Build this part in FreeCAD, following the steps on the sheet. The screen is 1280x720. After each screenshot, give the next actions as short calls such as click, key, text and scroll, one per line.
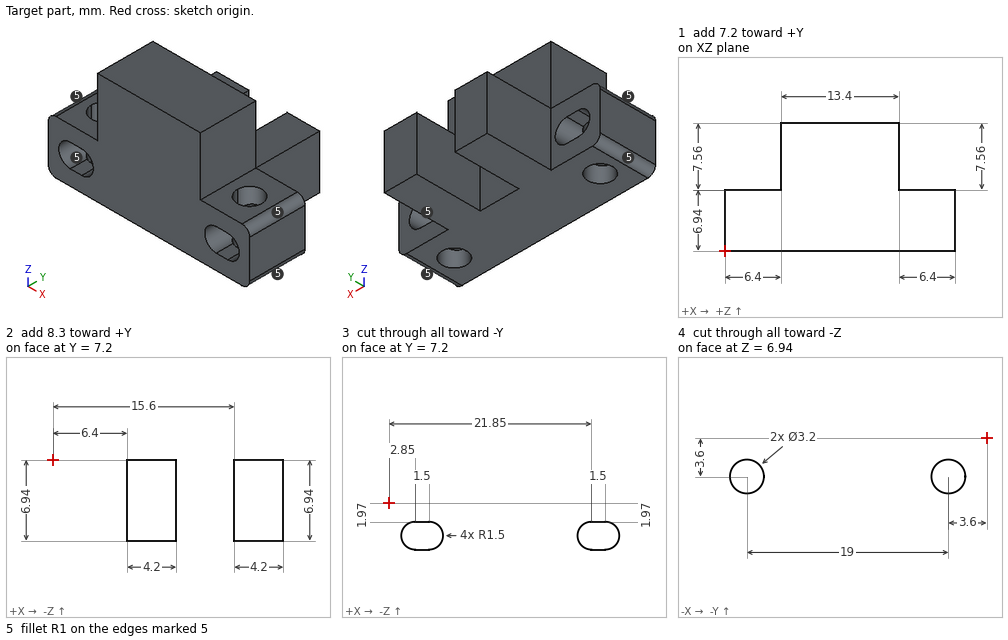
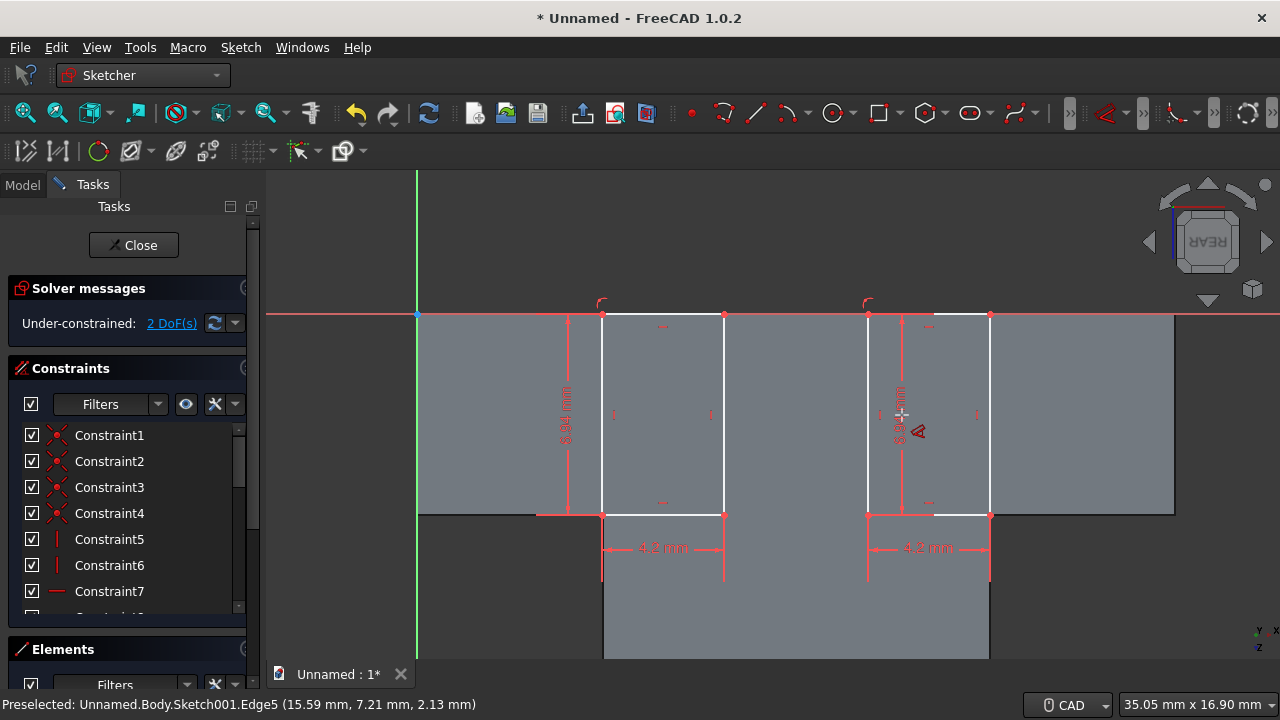
click(602, 314)
click(510, 280)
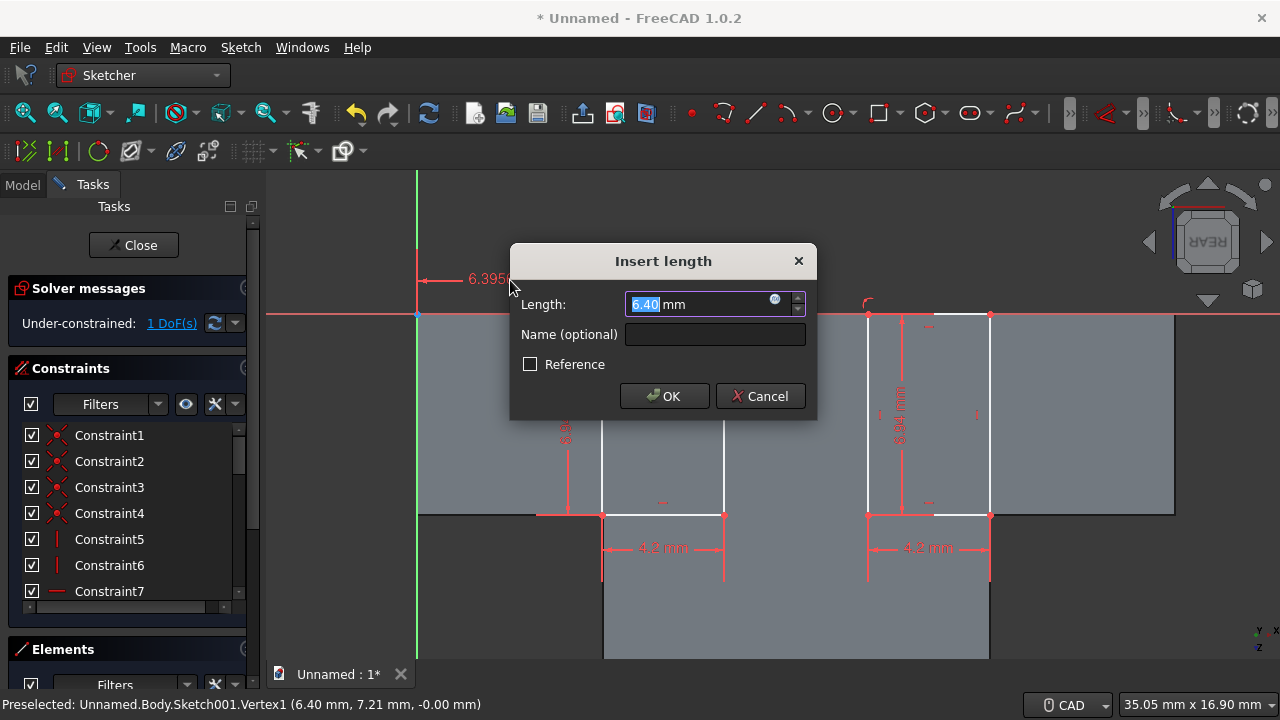
text(6.4)
key(Return)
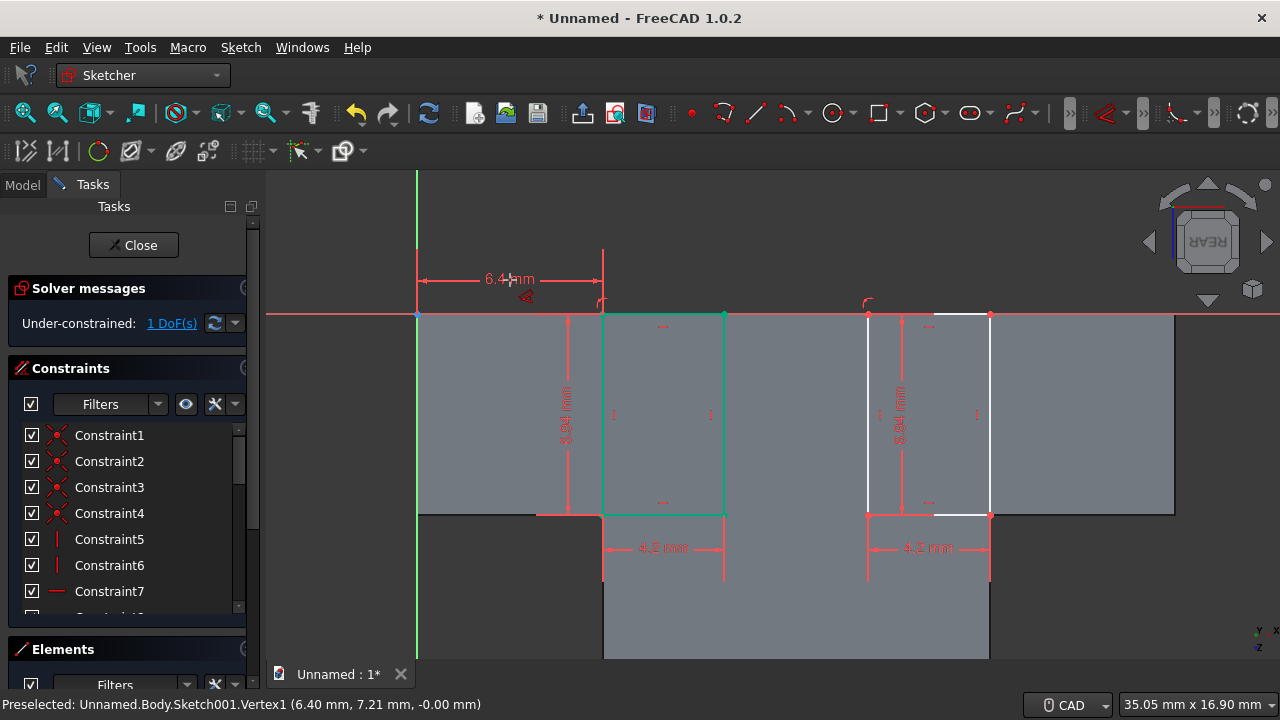
click(868, 314)
click(643, 280)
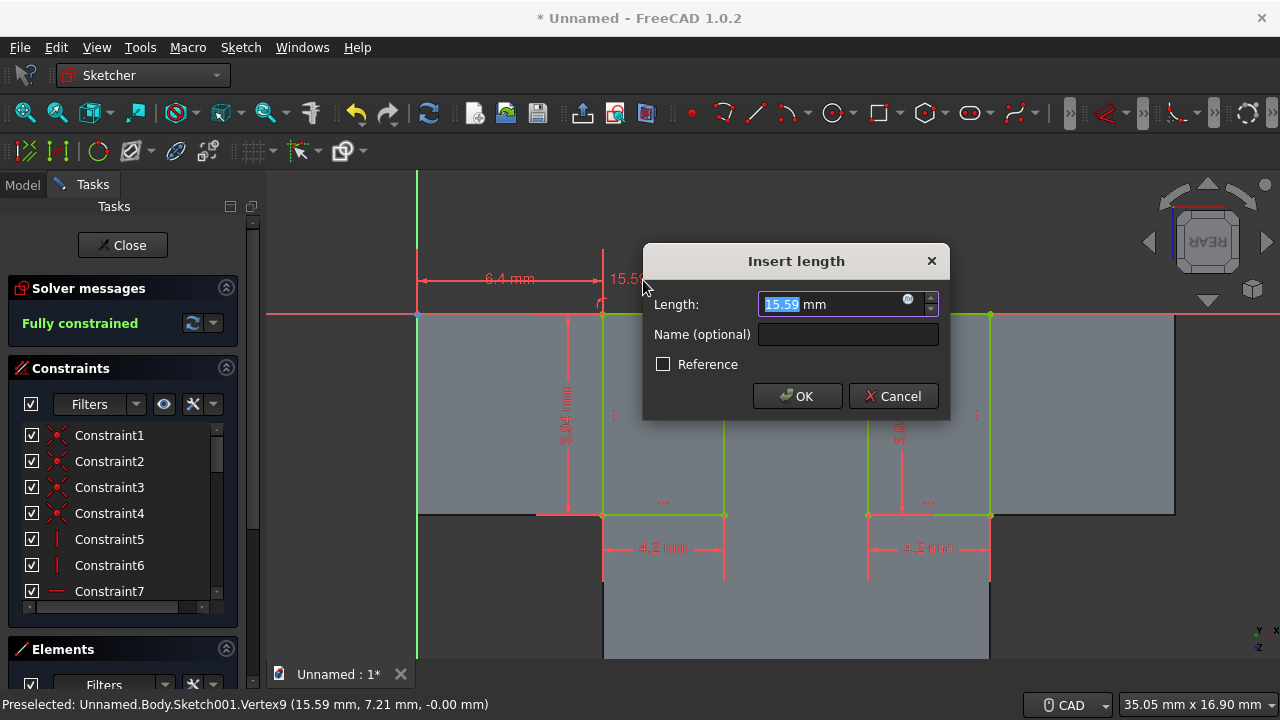
text(15.6)
key(Return)
key(Escape)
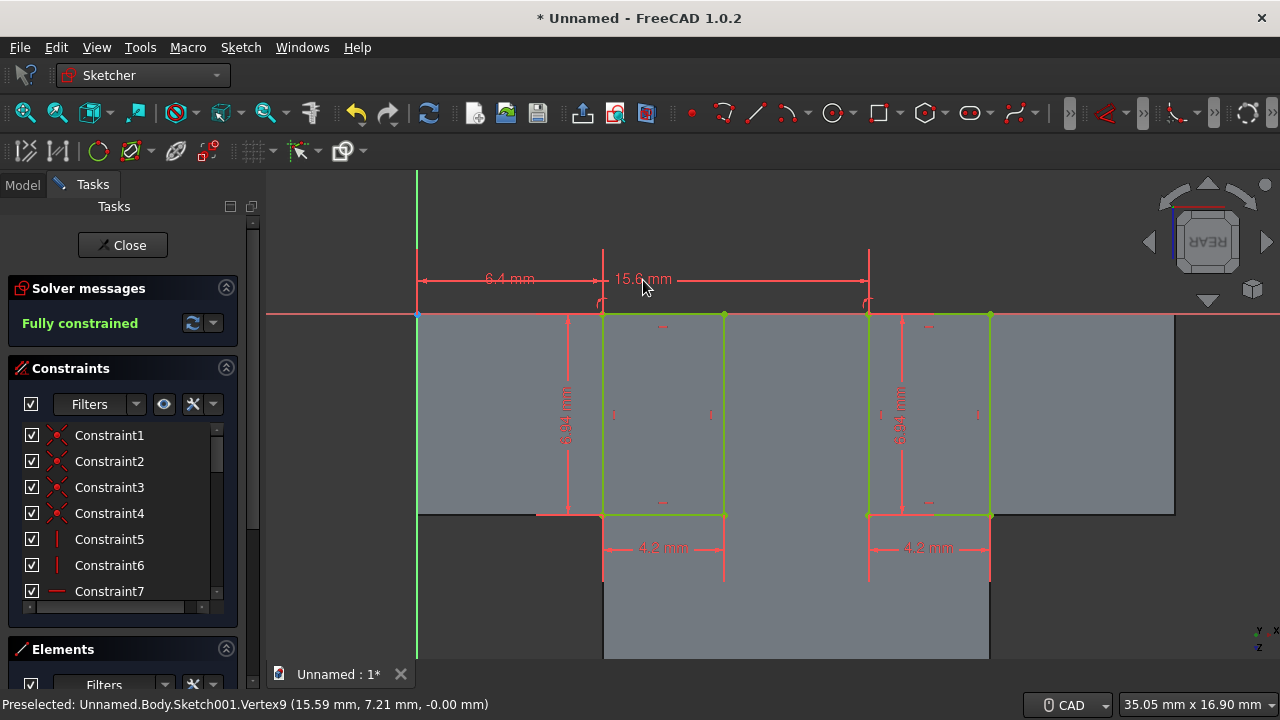
click(123, 245)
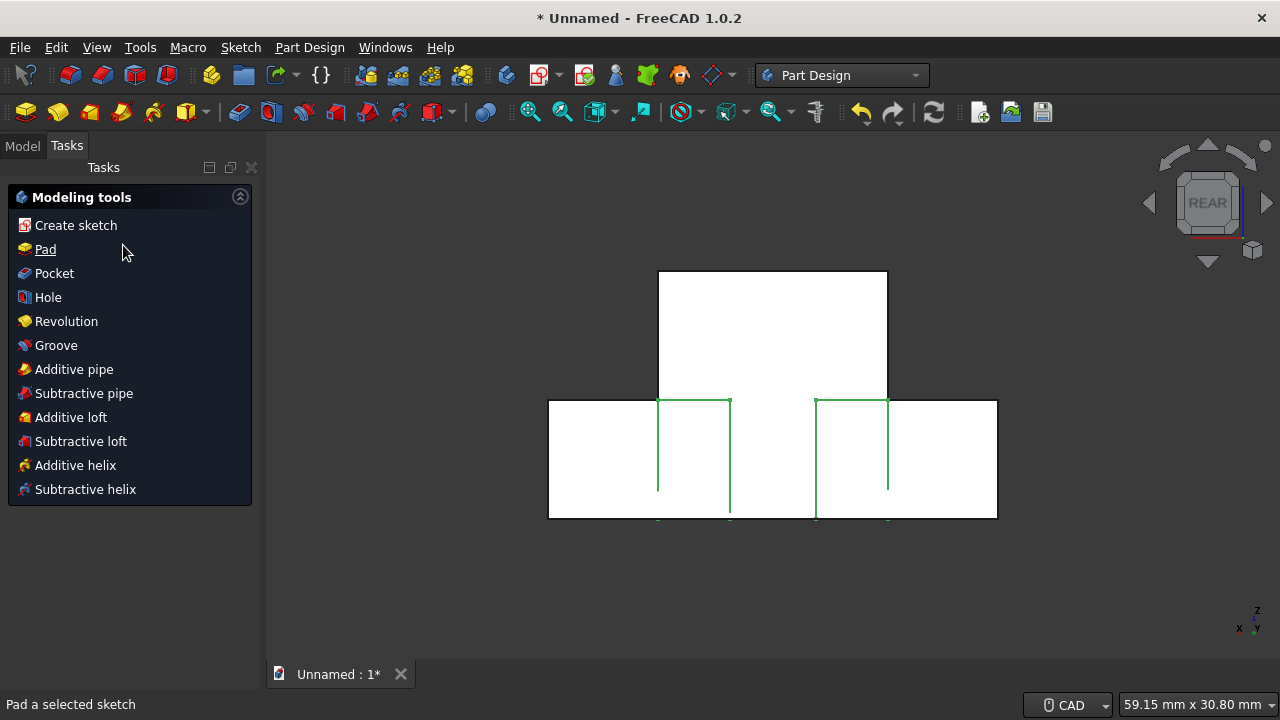
click(26, 112)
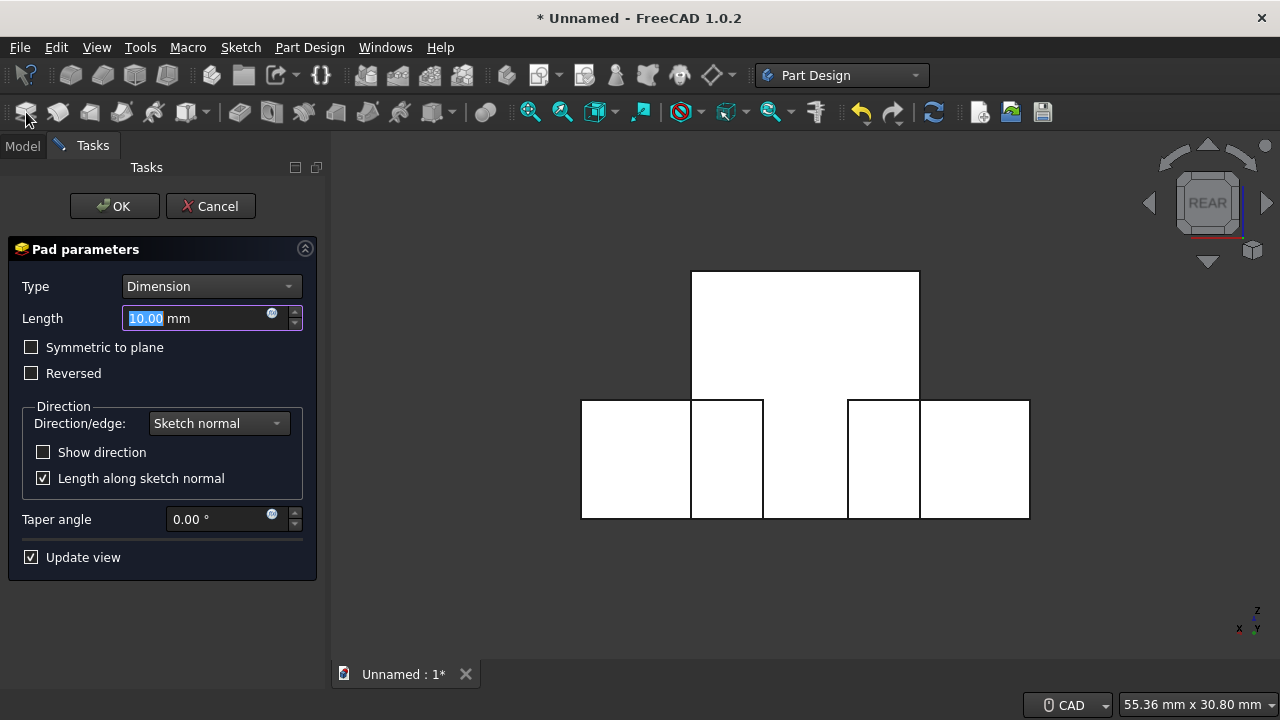
text(8.3)
key(Tab)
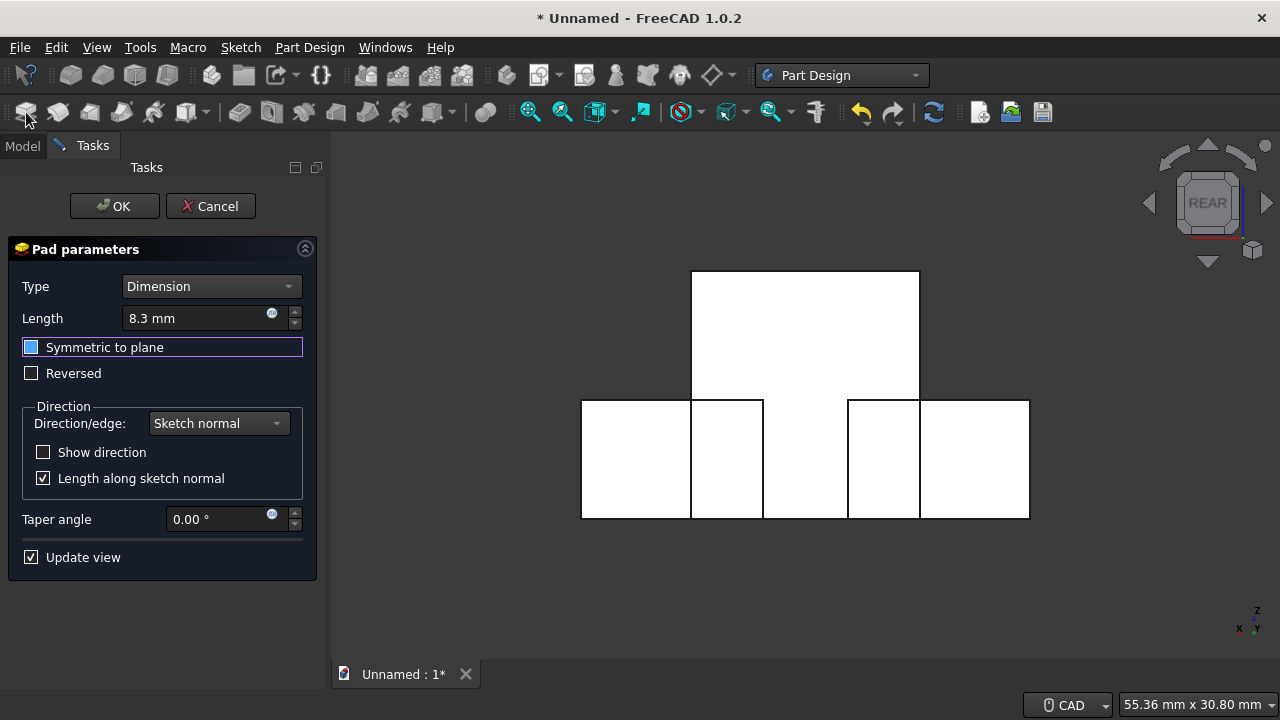
click(115, 206)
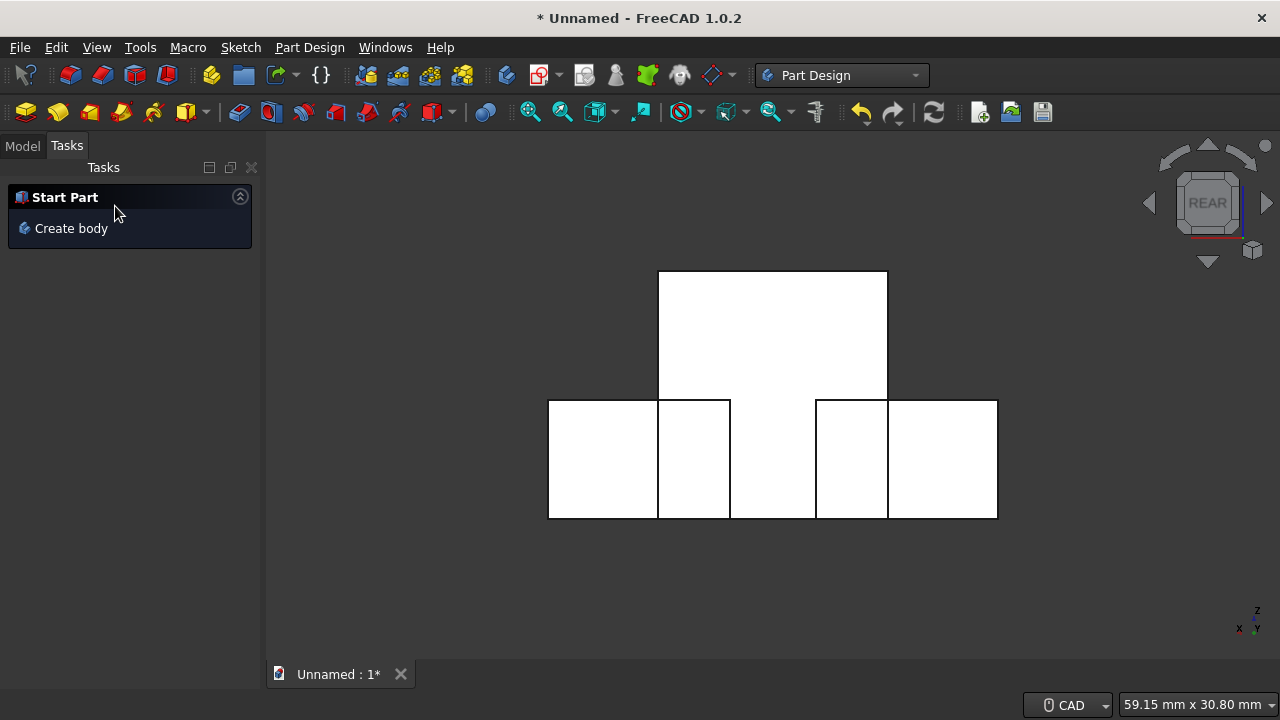
click(773, 358)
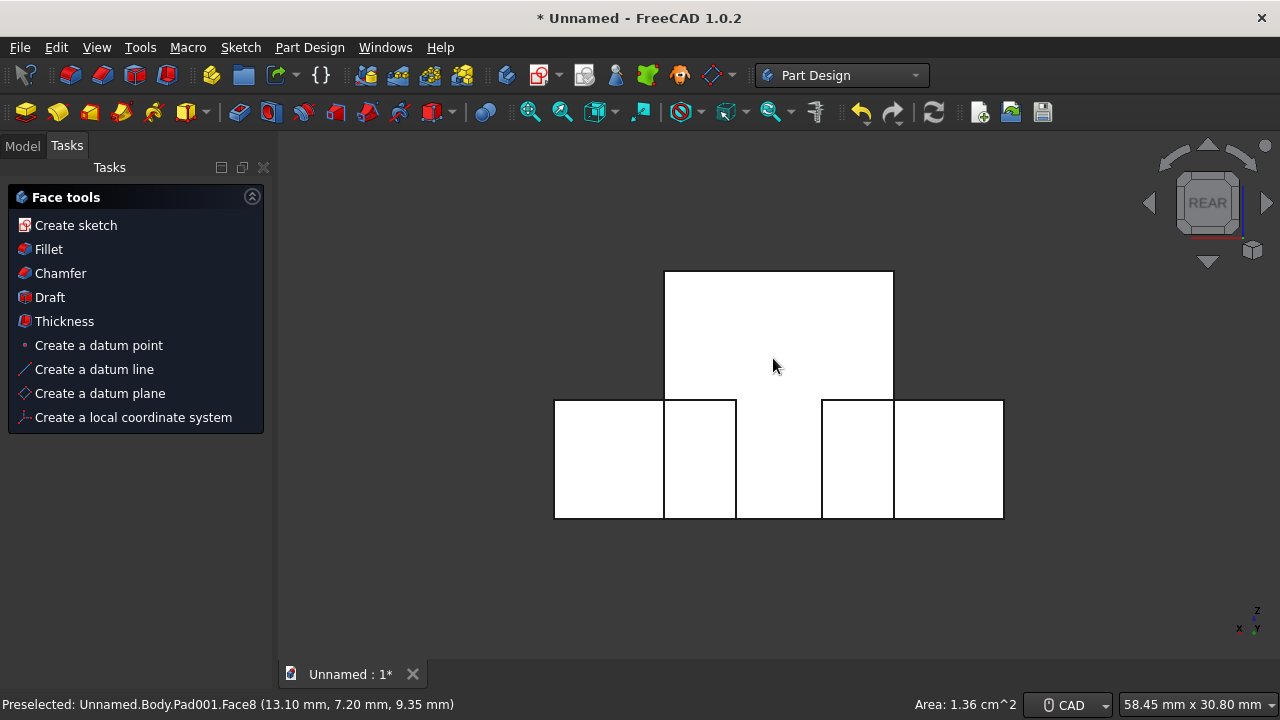
click(540, 76)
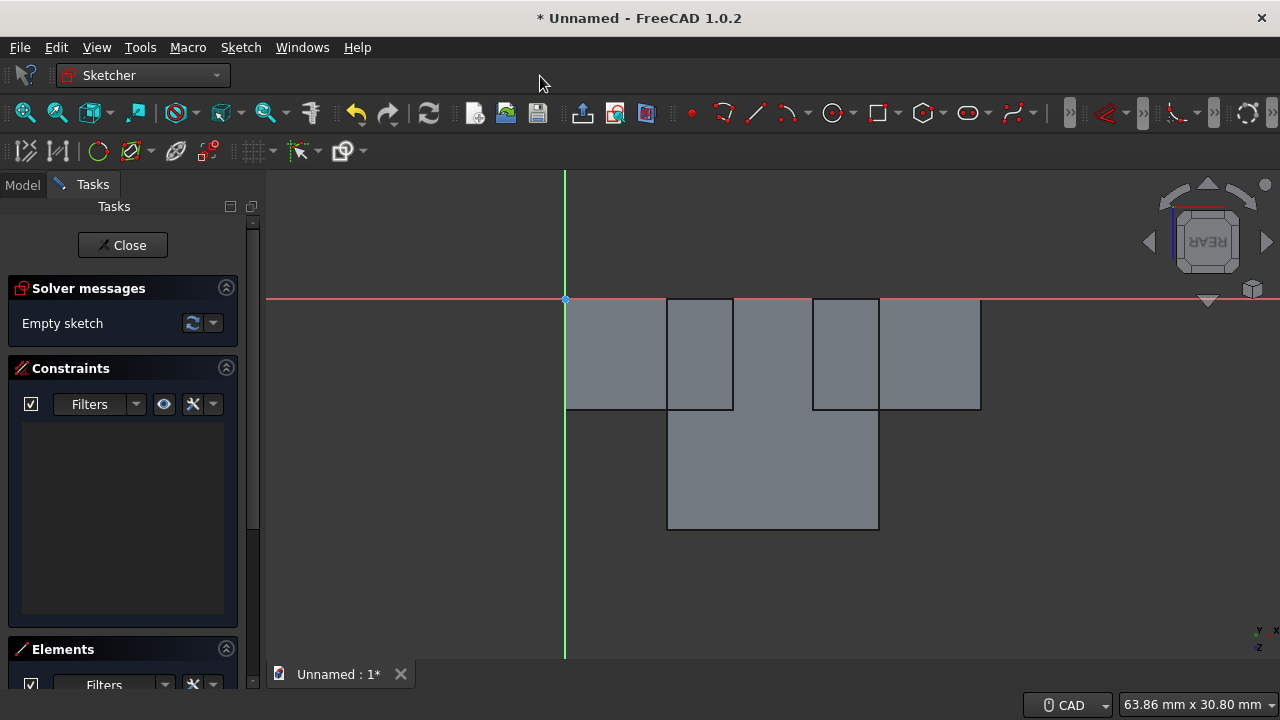
scroll(880, 198, up, 2)